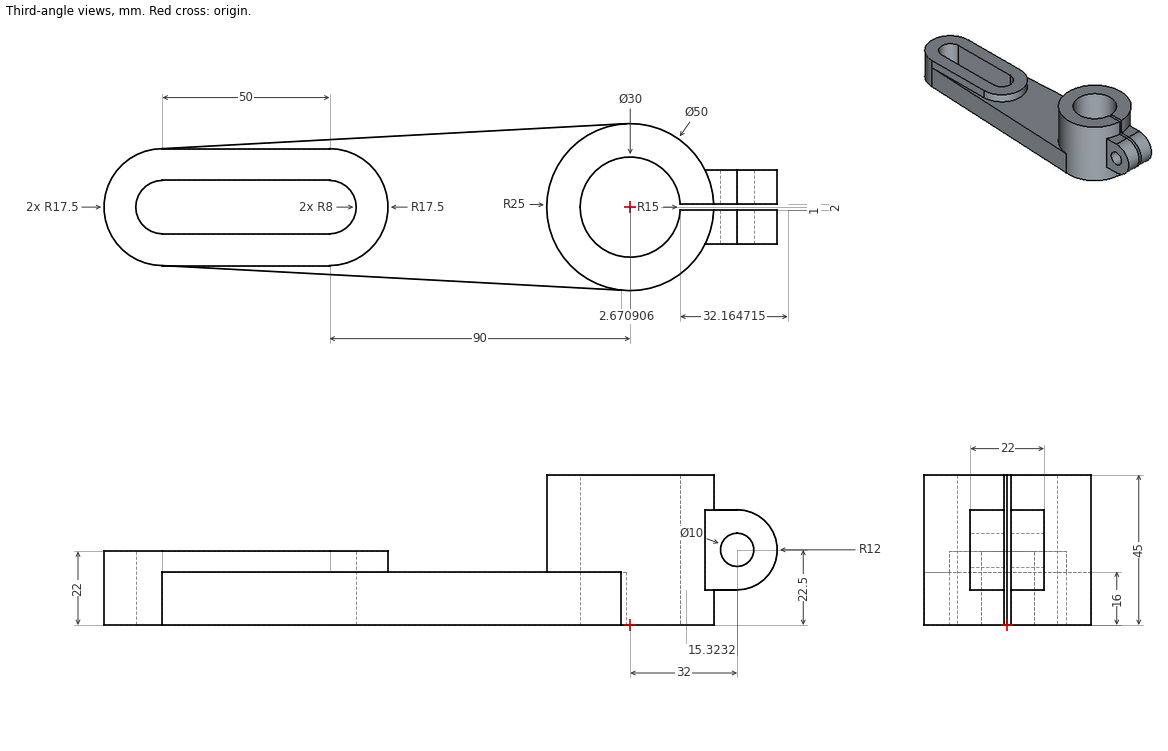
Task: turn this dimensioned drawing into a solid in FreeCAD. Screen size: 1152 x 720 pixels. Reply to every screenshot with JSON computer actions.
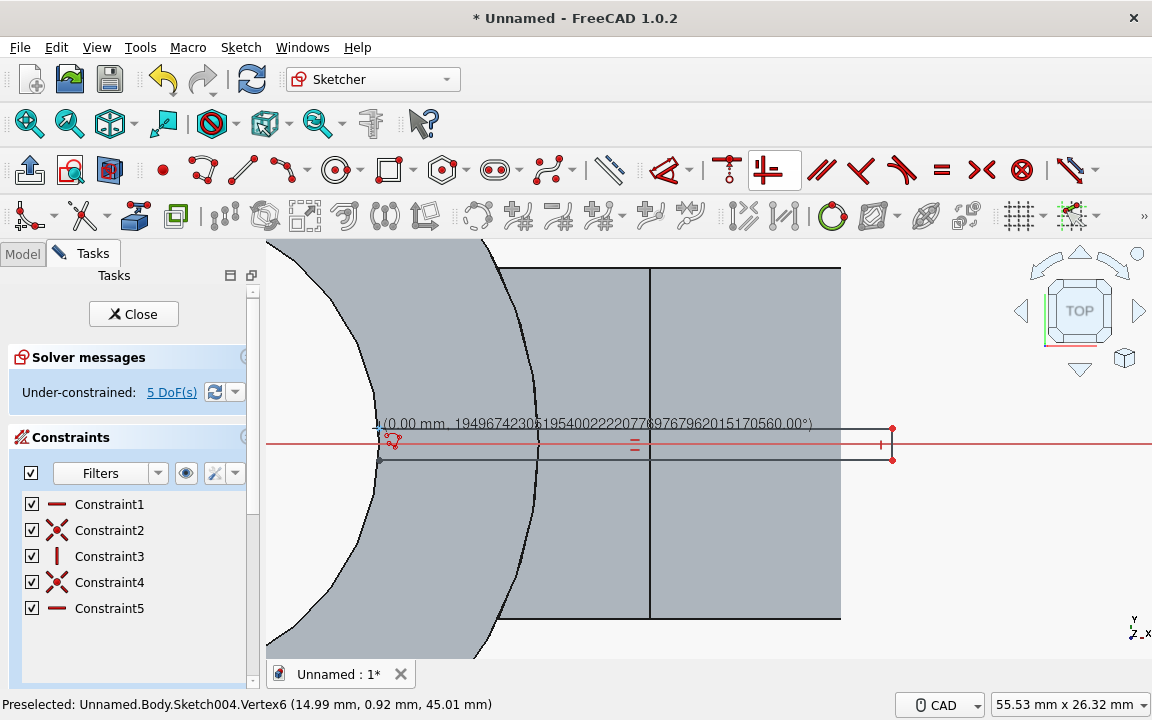
{"action": "left_click", "coordinate": [284, 170]}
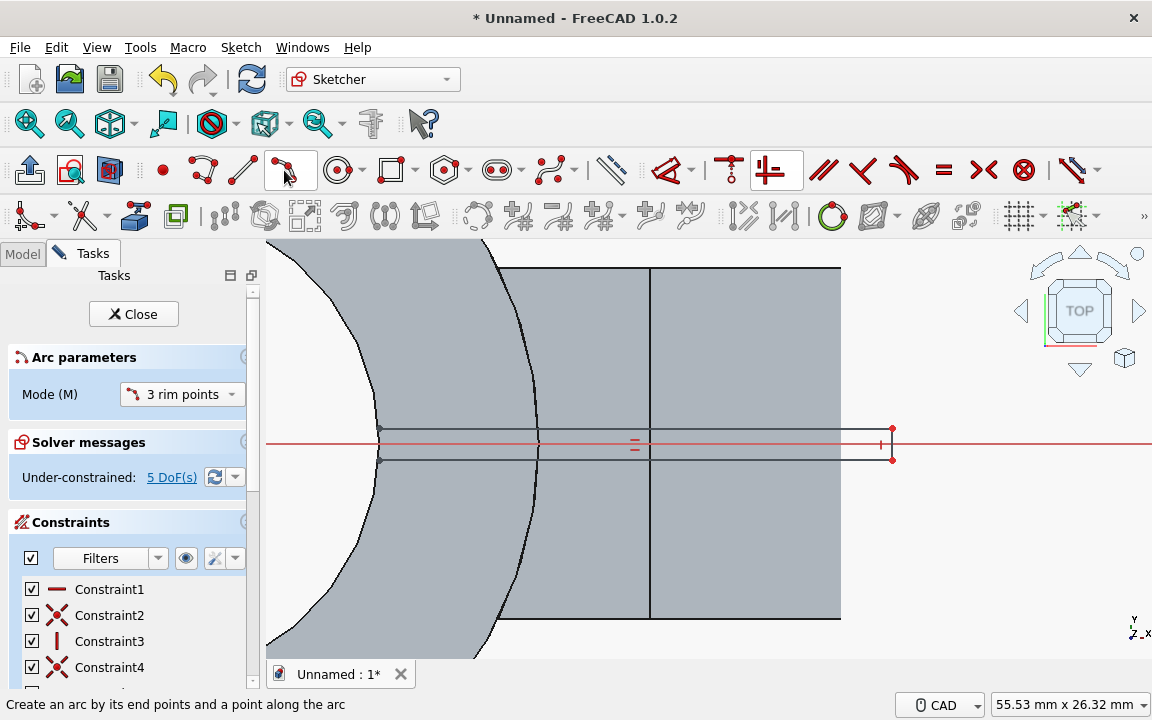
{"action": "left_click", "coordinate": [379, 429]}
{"action": "left_click", "coordinate": [379, 460]}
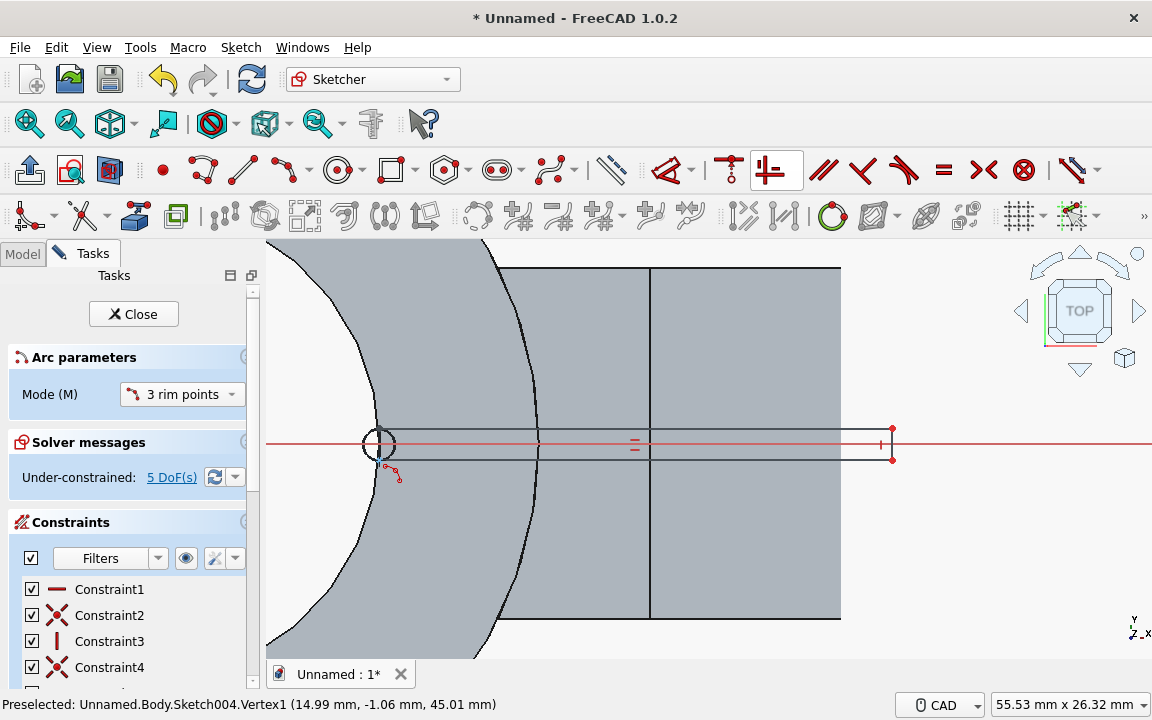
{"action": "scroll", "coordinate": [379, 447], "scroll_direction": "up", "scroll_amount": 18}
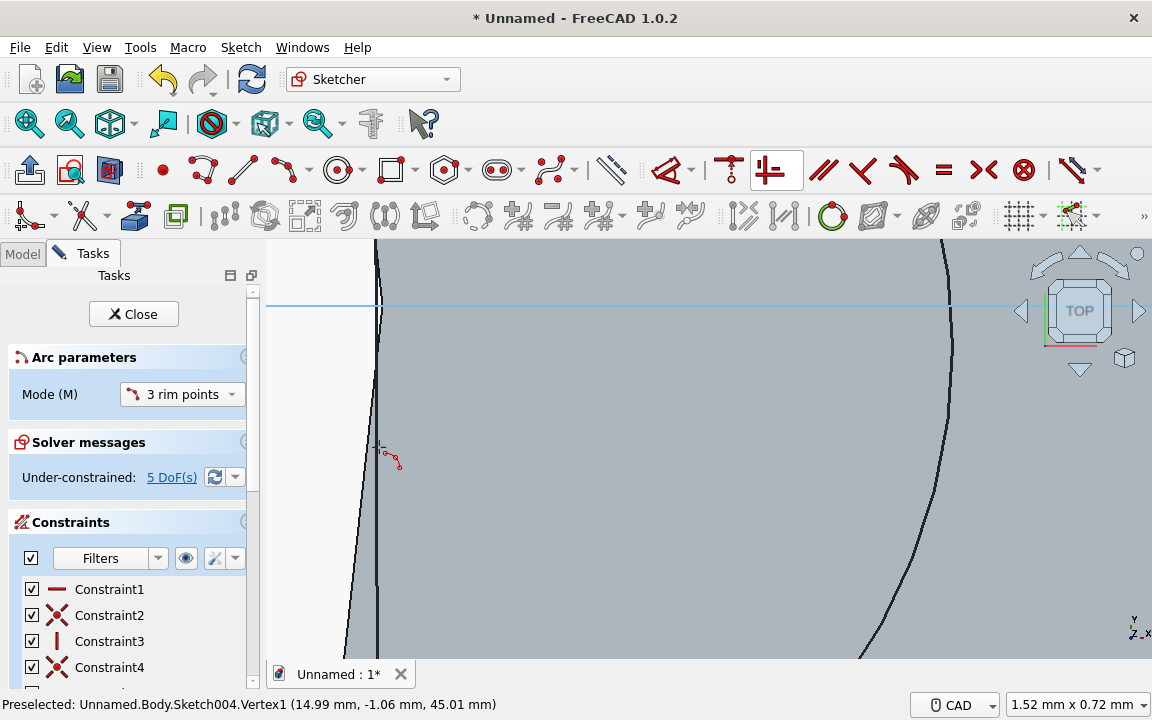
{"action": "left_click", "coordinate": [382, 422]}
{"action": "key", "text": "Escape"}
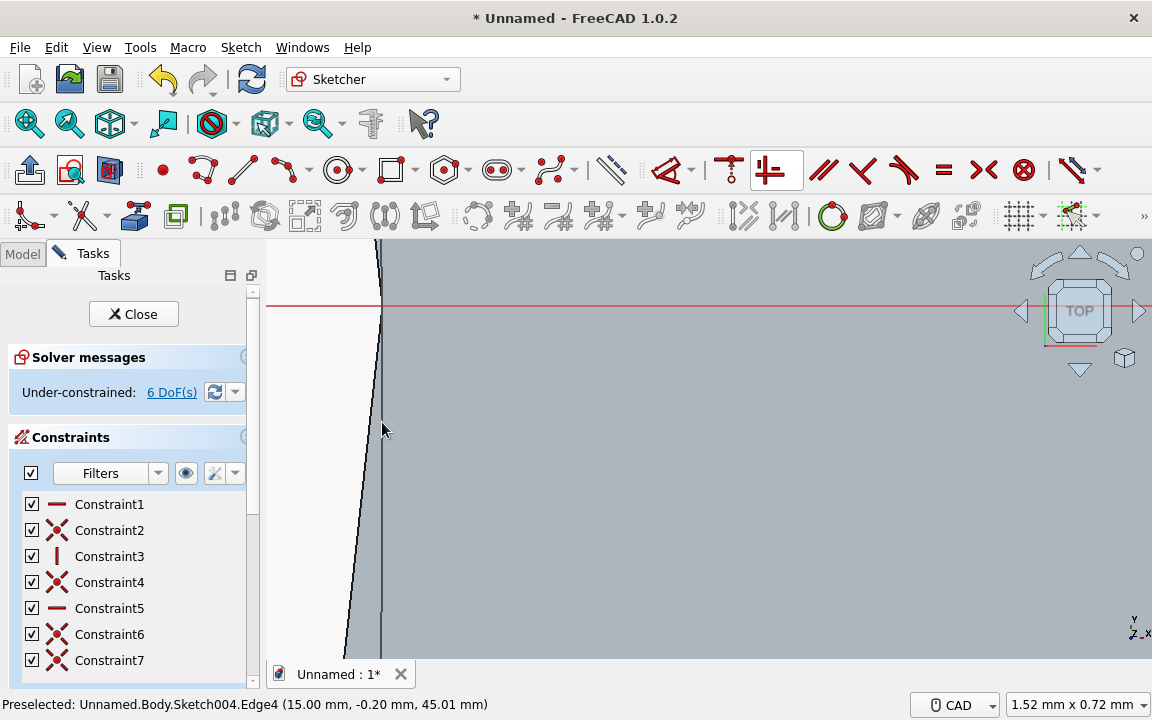
{"action": "scroll", "coordinate": [640, 449], "scroll_direction": "down", "scroll_amount": 15}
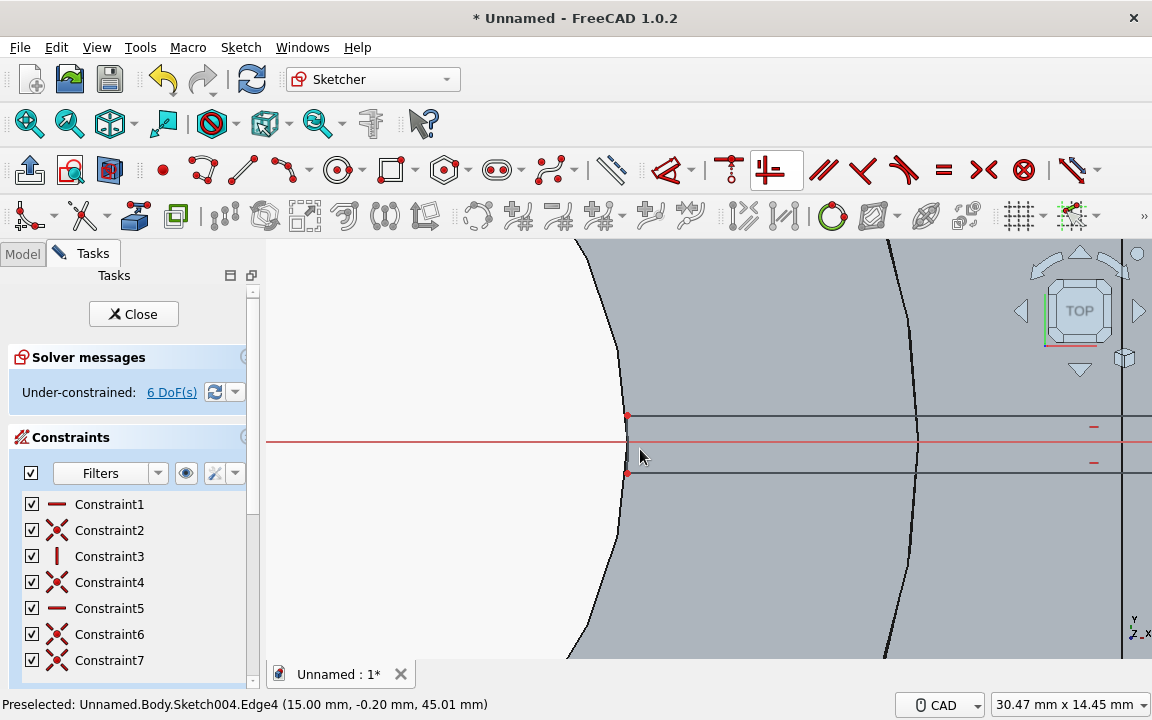
{"action": "scroll", "coordinate": [503, 453], "scroll_direction": "down", "scroll_amount": 5}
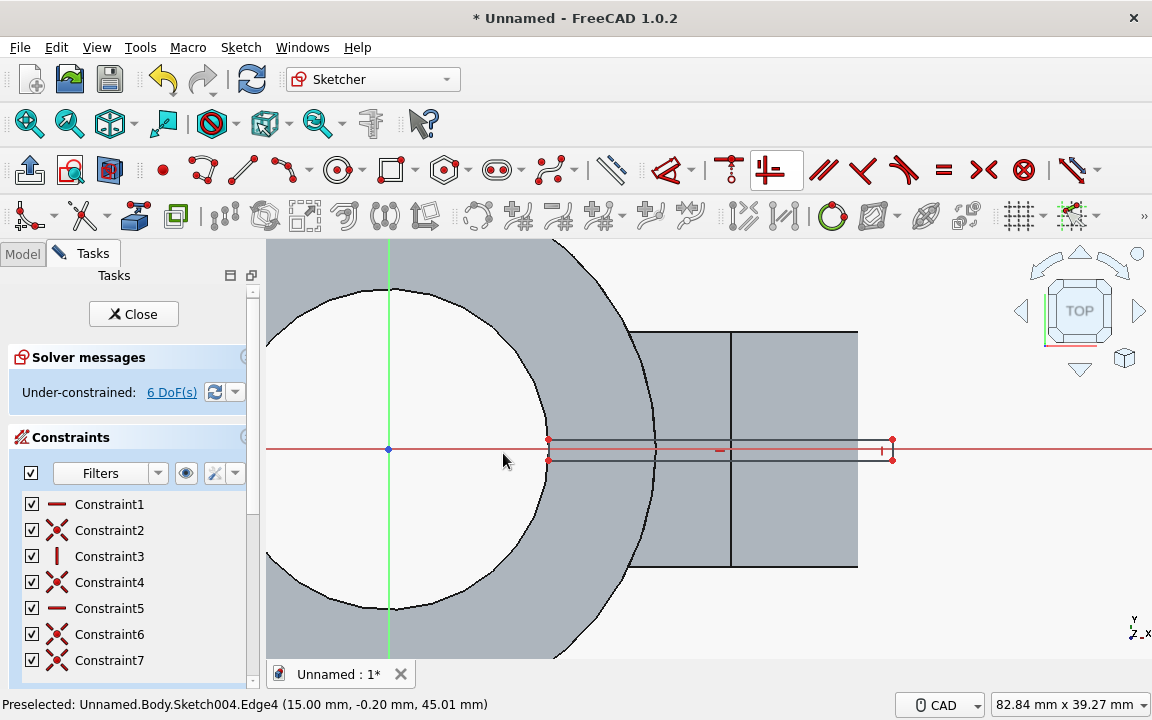
{"action": "scroll", "coordinate": [835, 448], "scroll_direction": "down", "scroll_amount": 2}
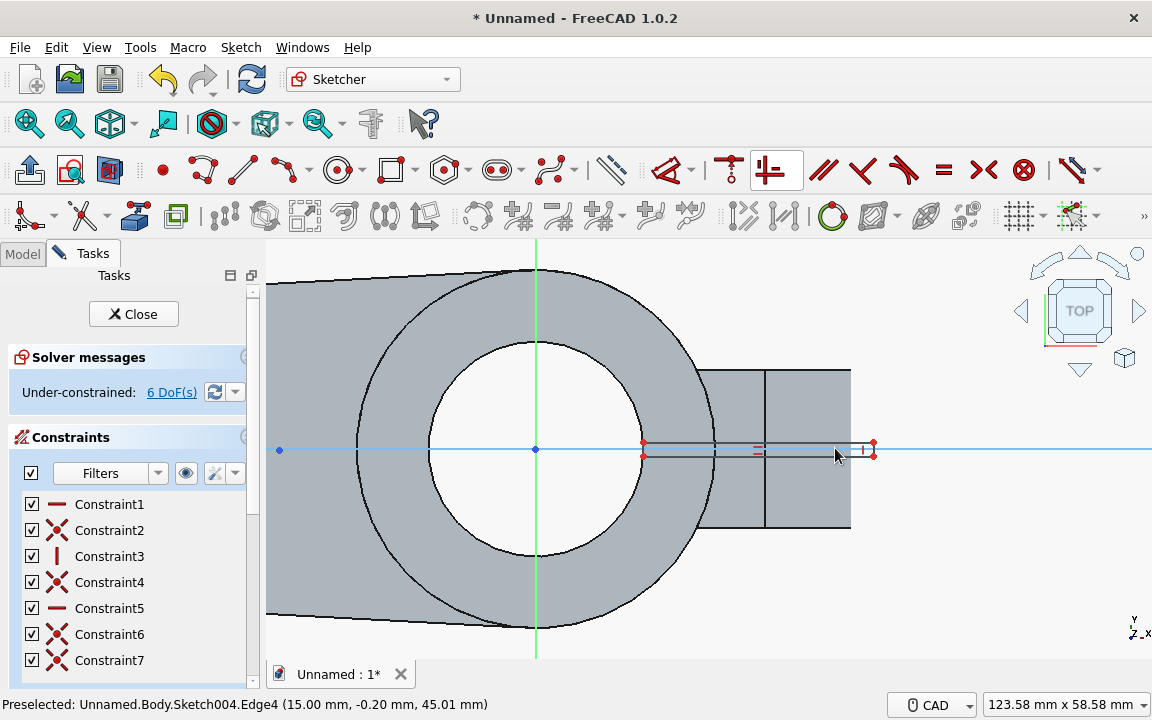
{"action": "left_click_drag", "start_coordinate": [270, 439], "coordinate": [546, 461]}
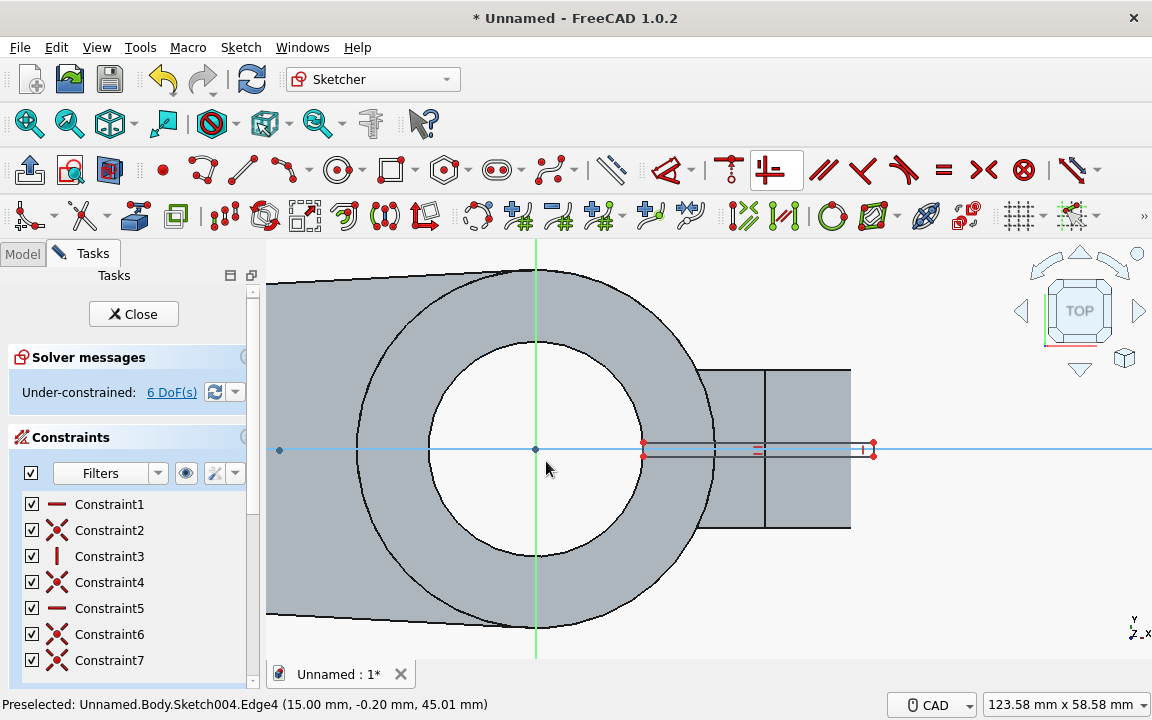
{"action": "left_click", "coordinate": [730, 170]}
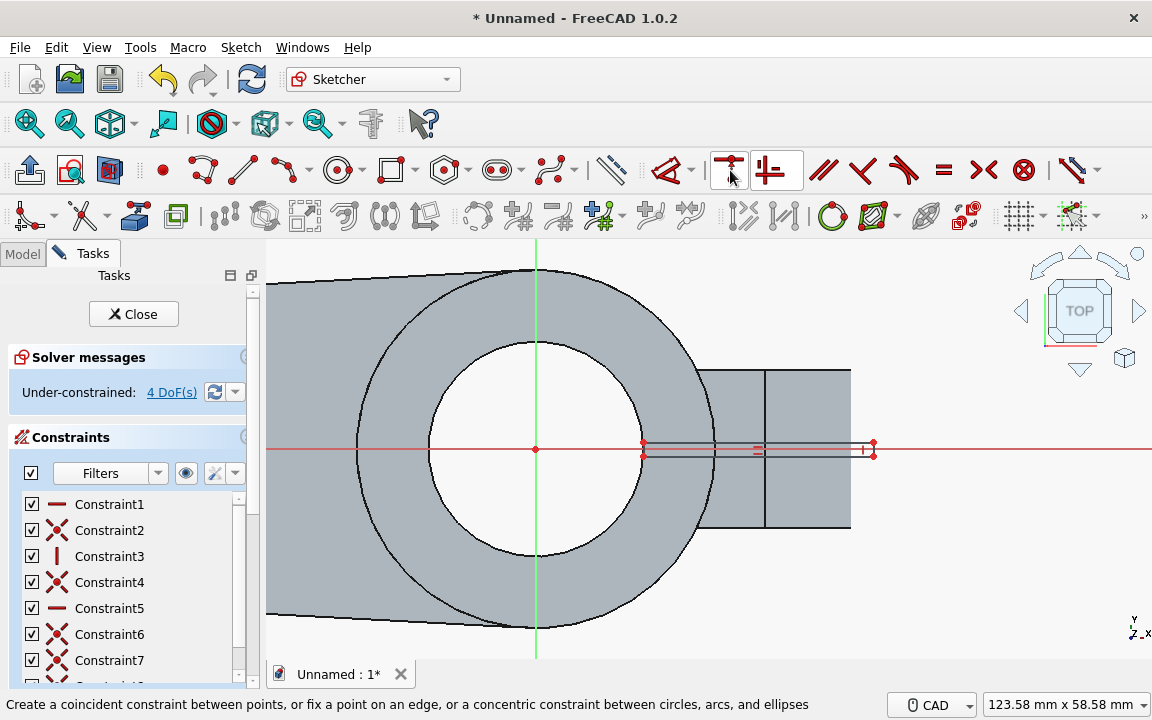
{"action": "left_click", "coordinate": [666, 170]}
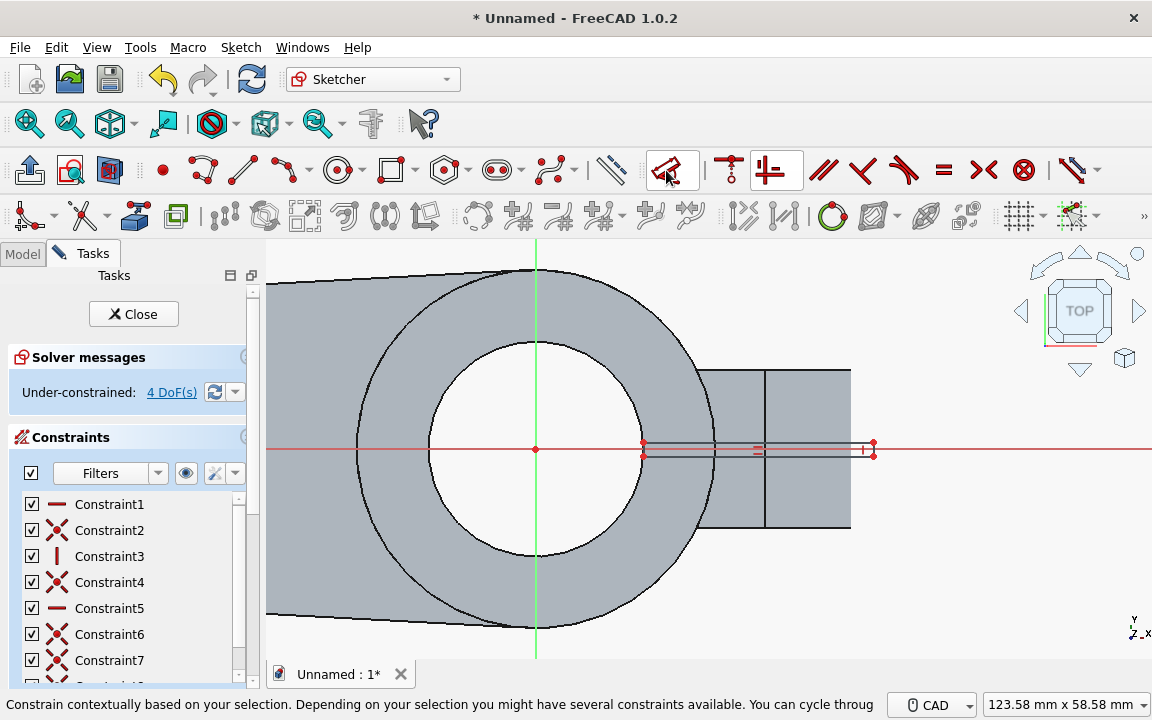
{"action": "scroll", "coordinate": [644, 450], "scroll_direction": "up", "scroll_amount": 4}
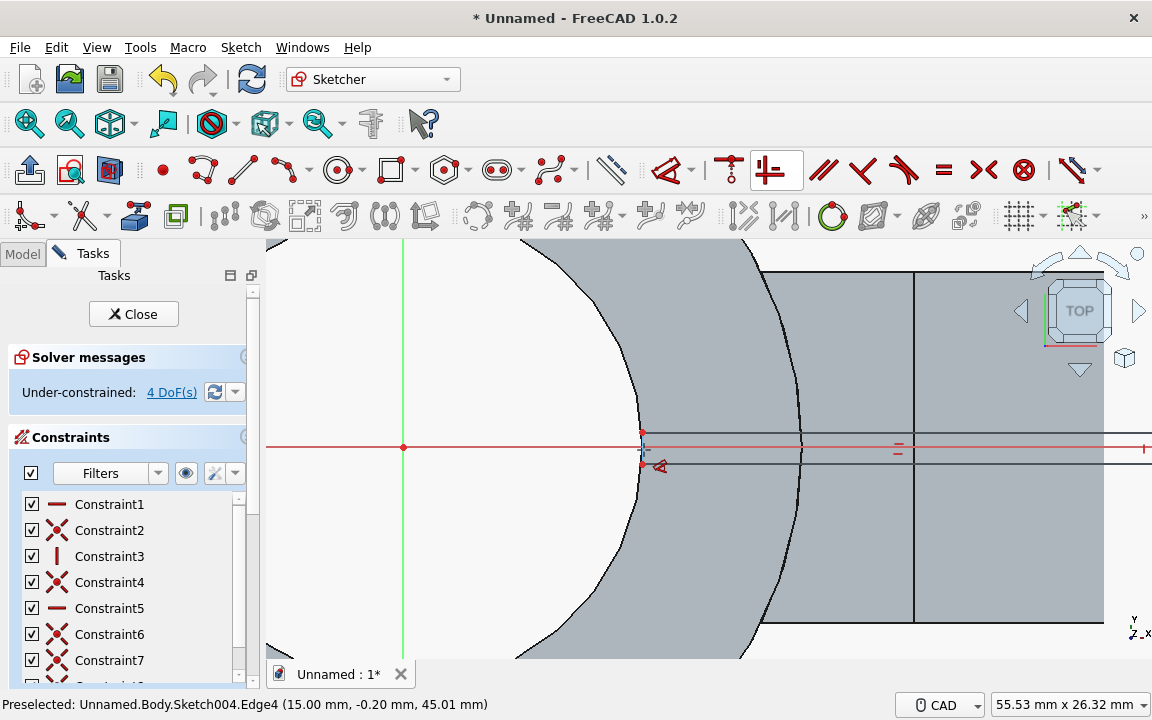
{"action": "left_click", "coordinate": [643, 449]}
{"action": "left_click", "coordinate": [641, 579]}